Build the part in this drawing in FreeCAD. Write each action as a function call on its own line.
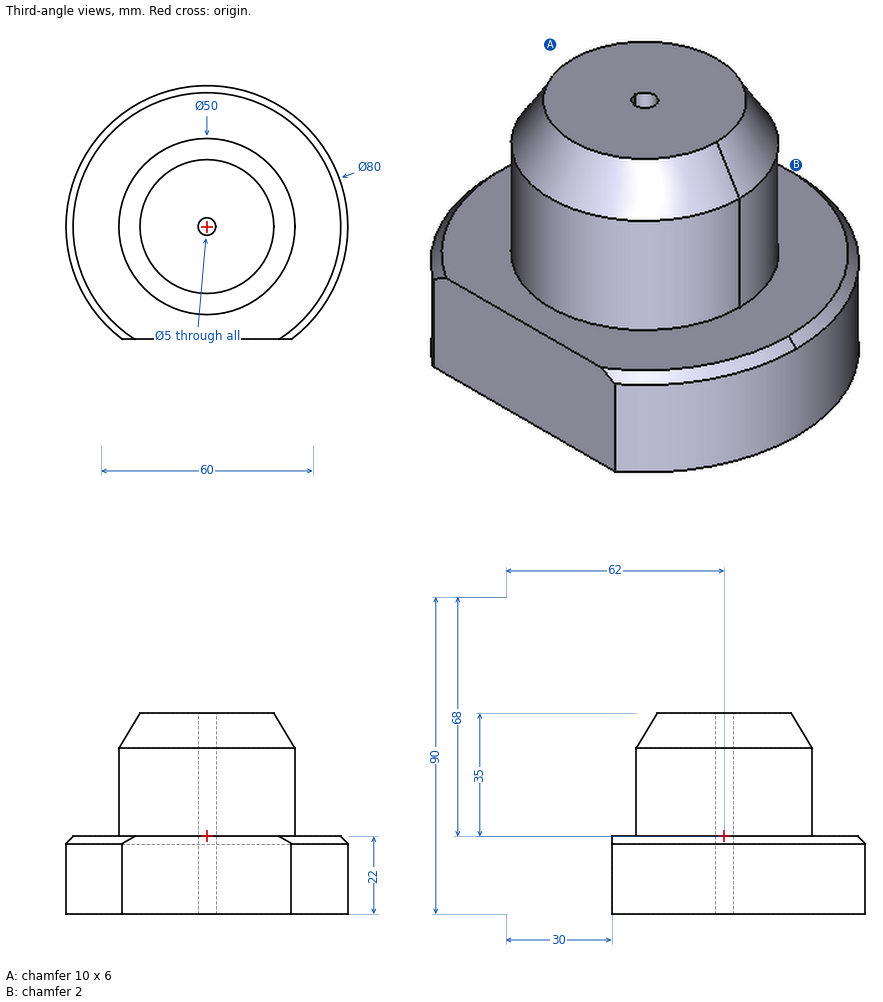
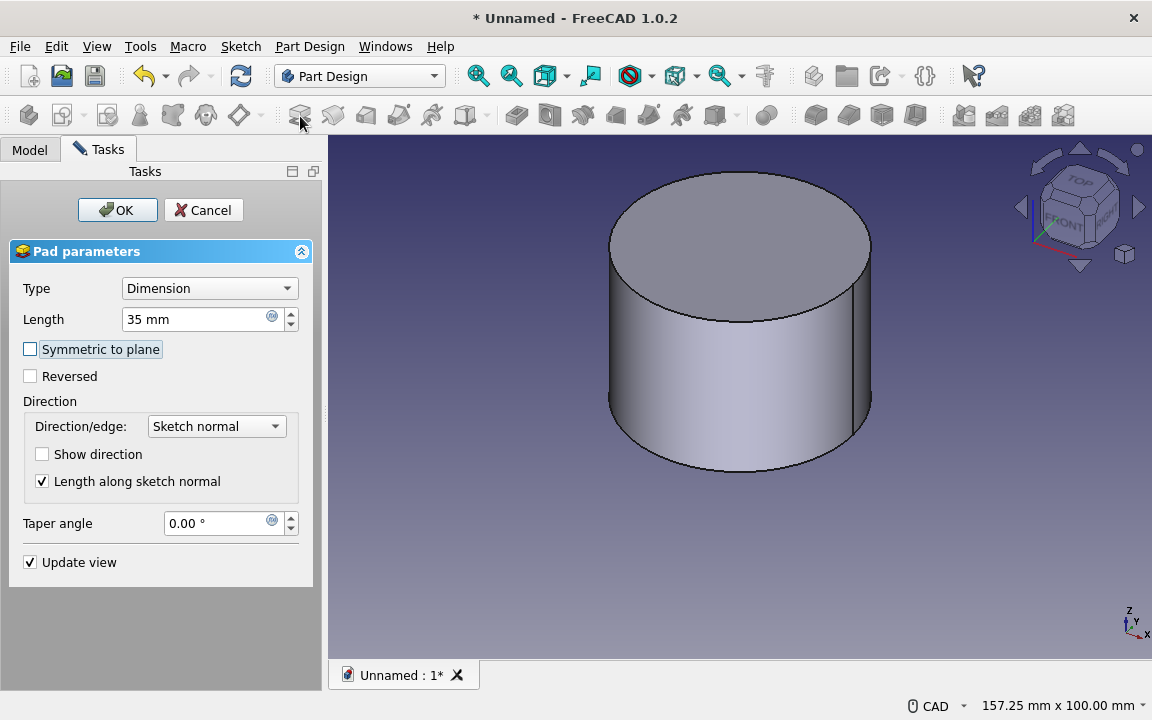
click(118, 210)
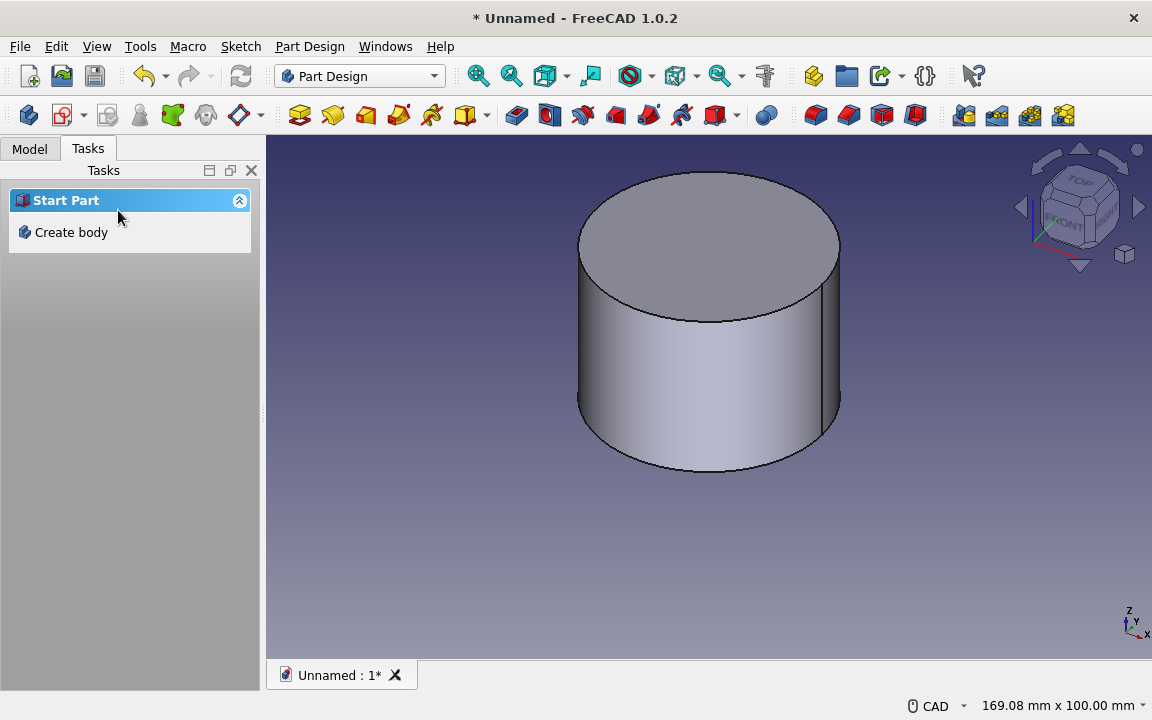
click(579, 254)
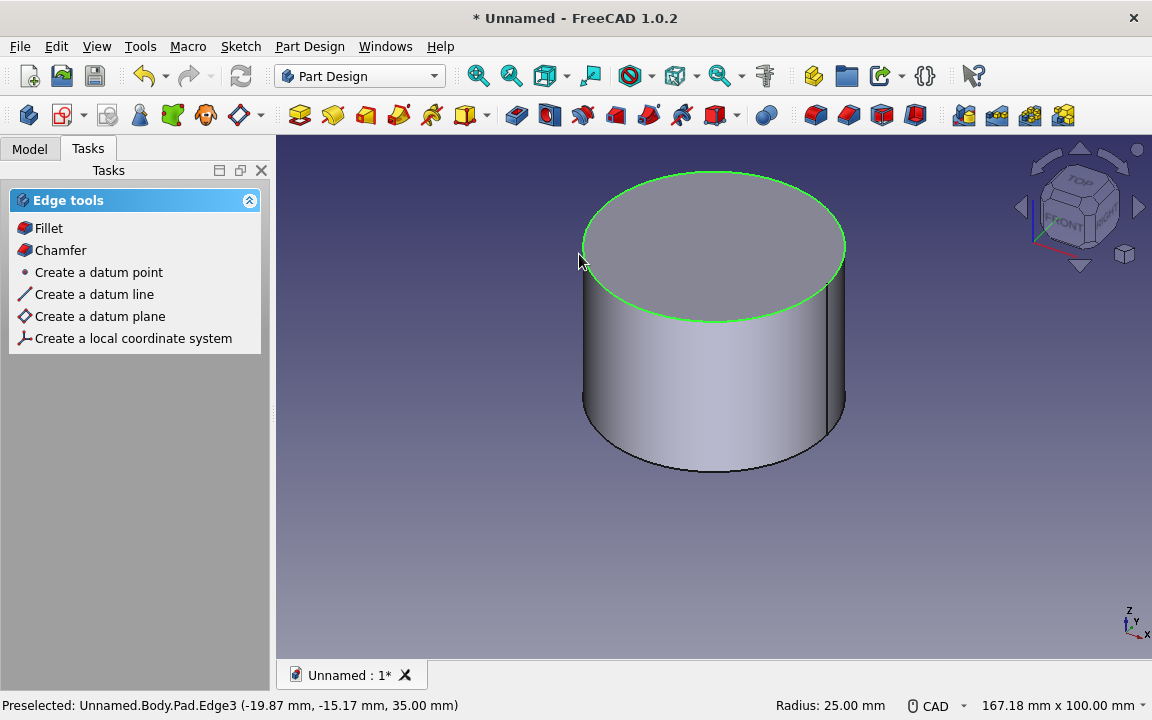
click(849, 116)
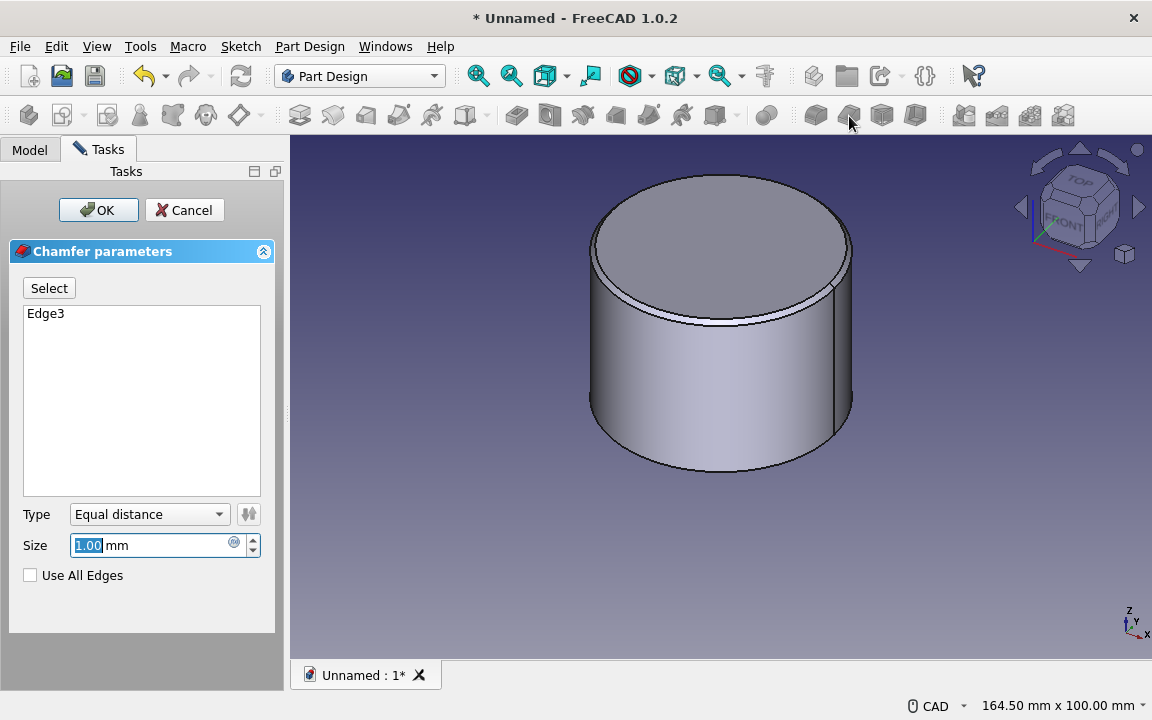
text(10)
key(Tab)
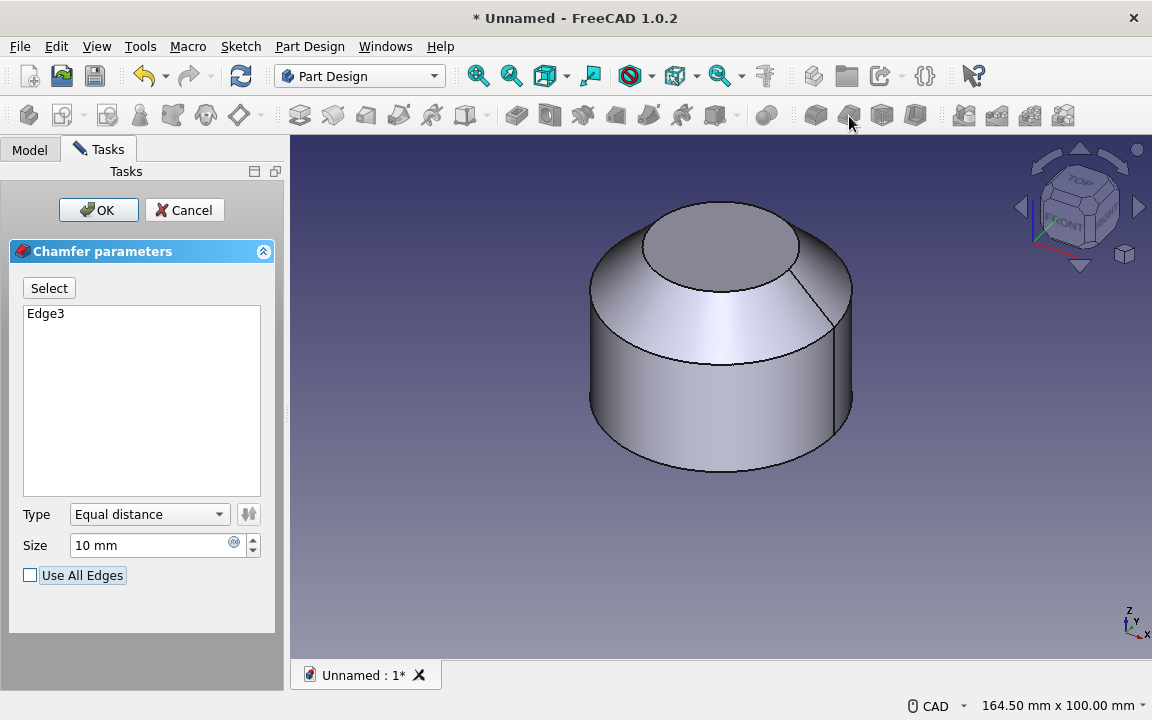
click(150, 514)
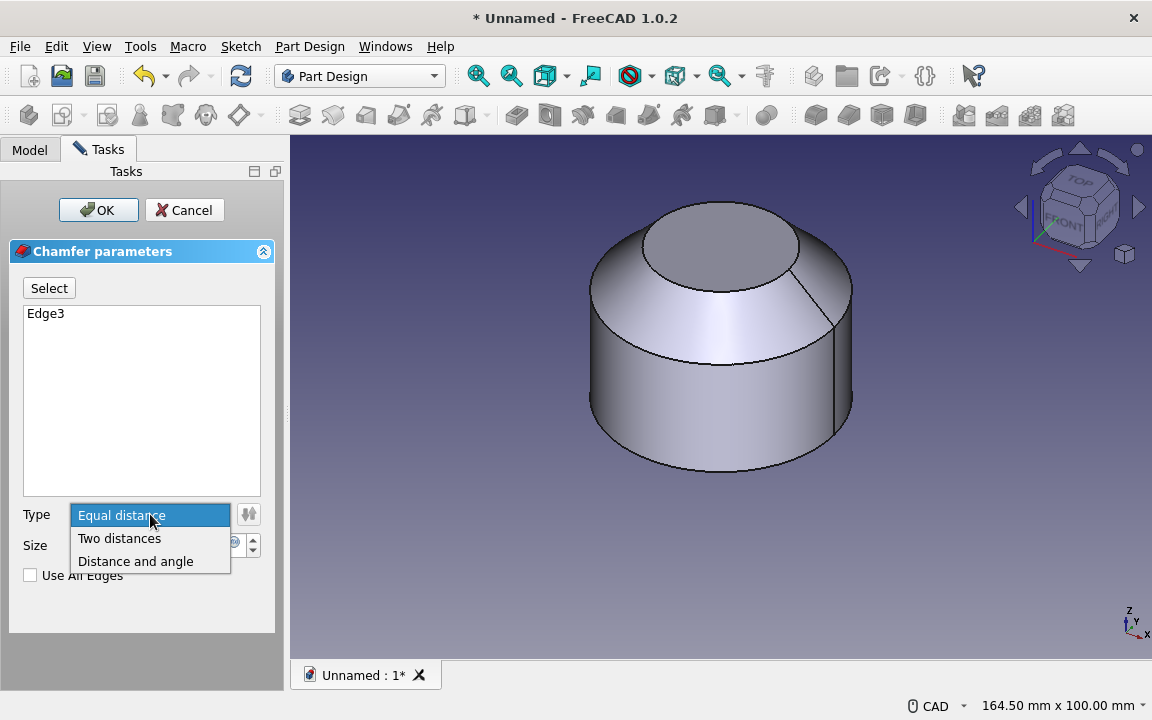
click(148, 538)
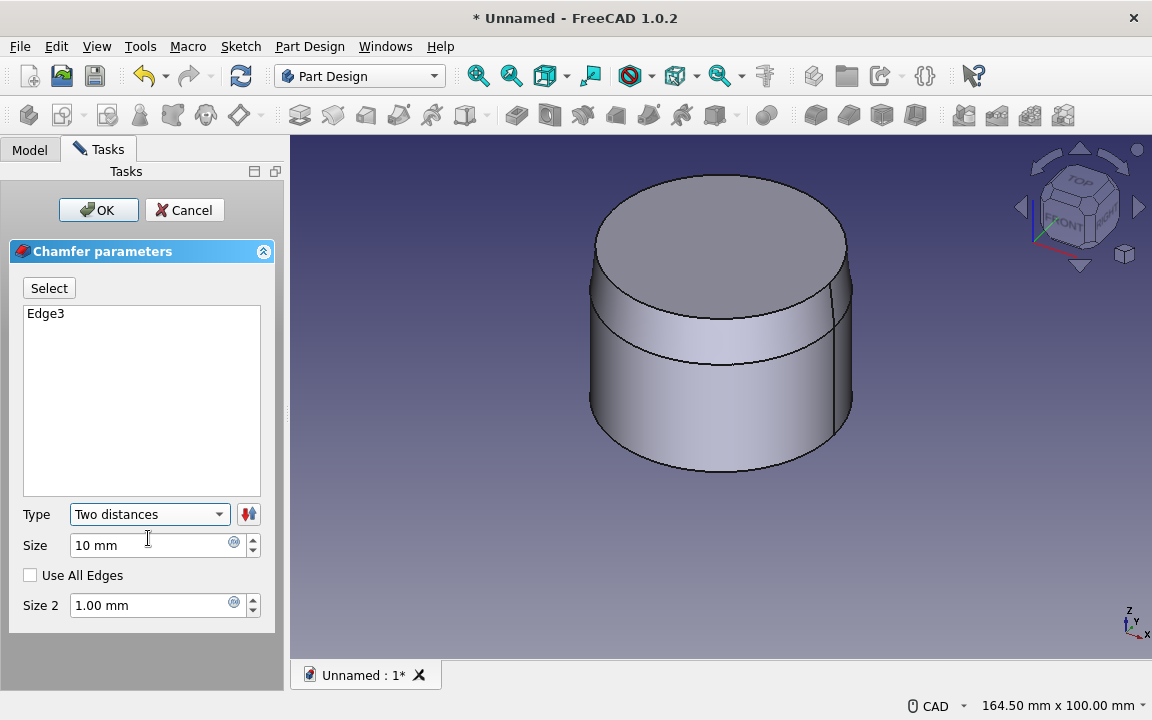
triple_click(158, 606)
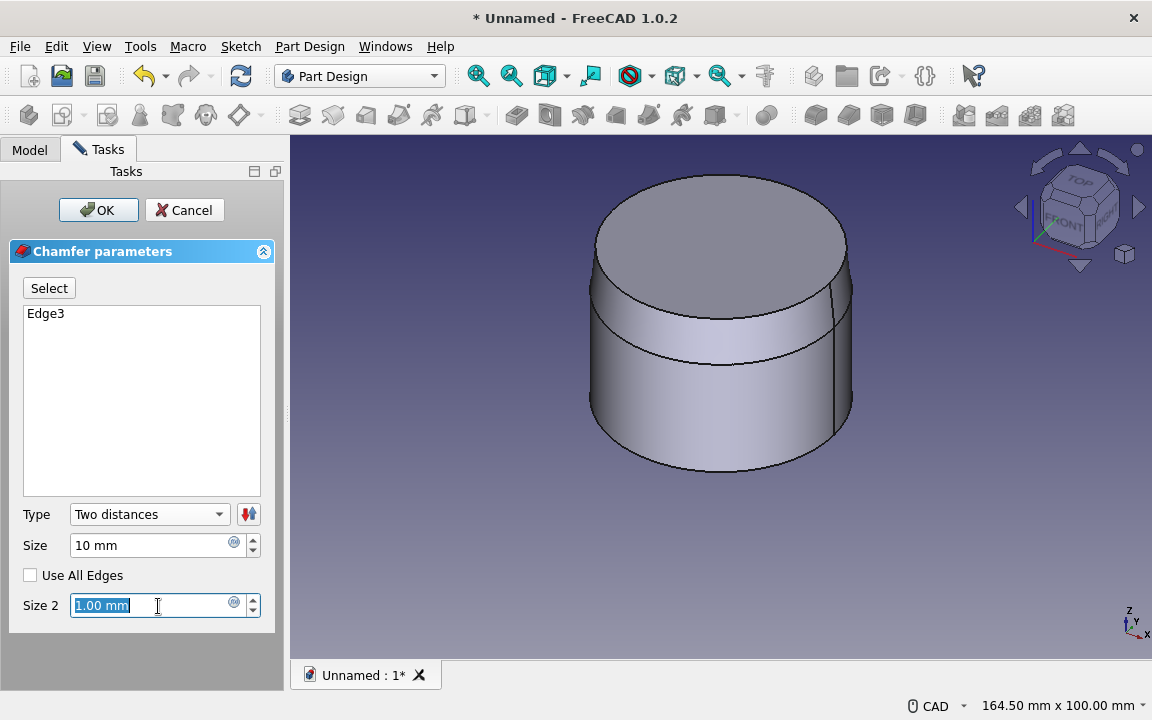
text(6)
key(Tab)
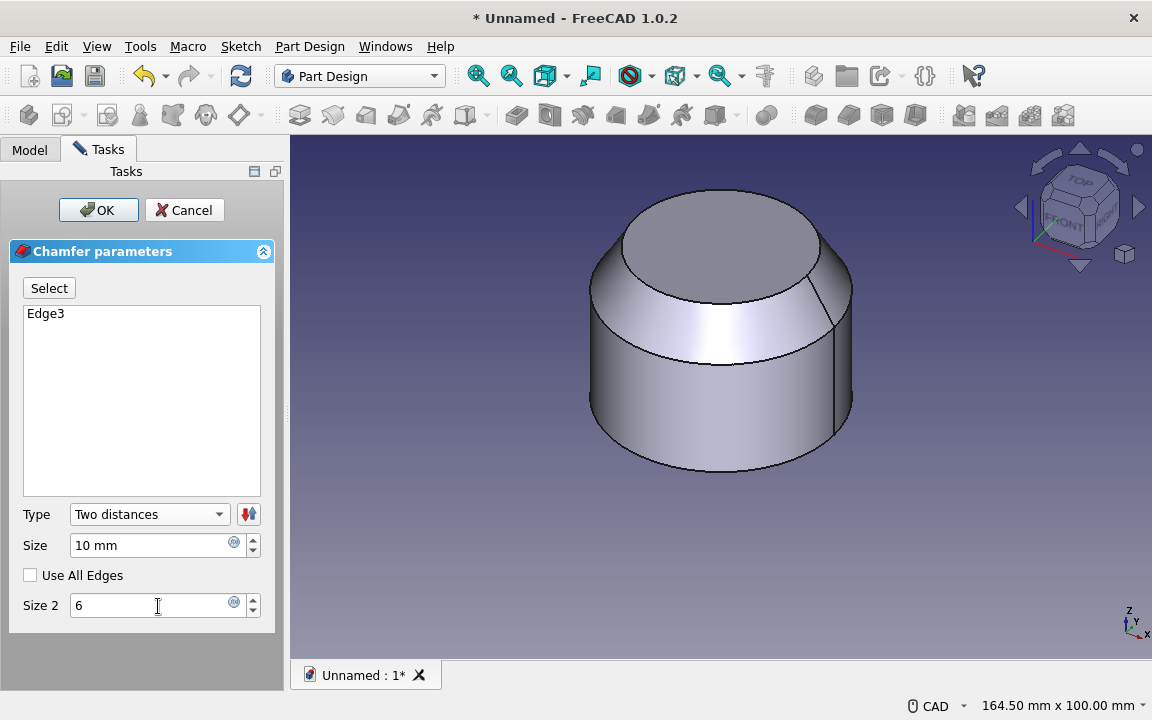
click(99, 210)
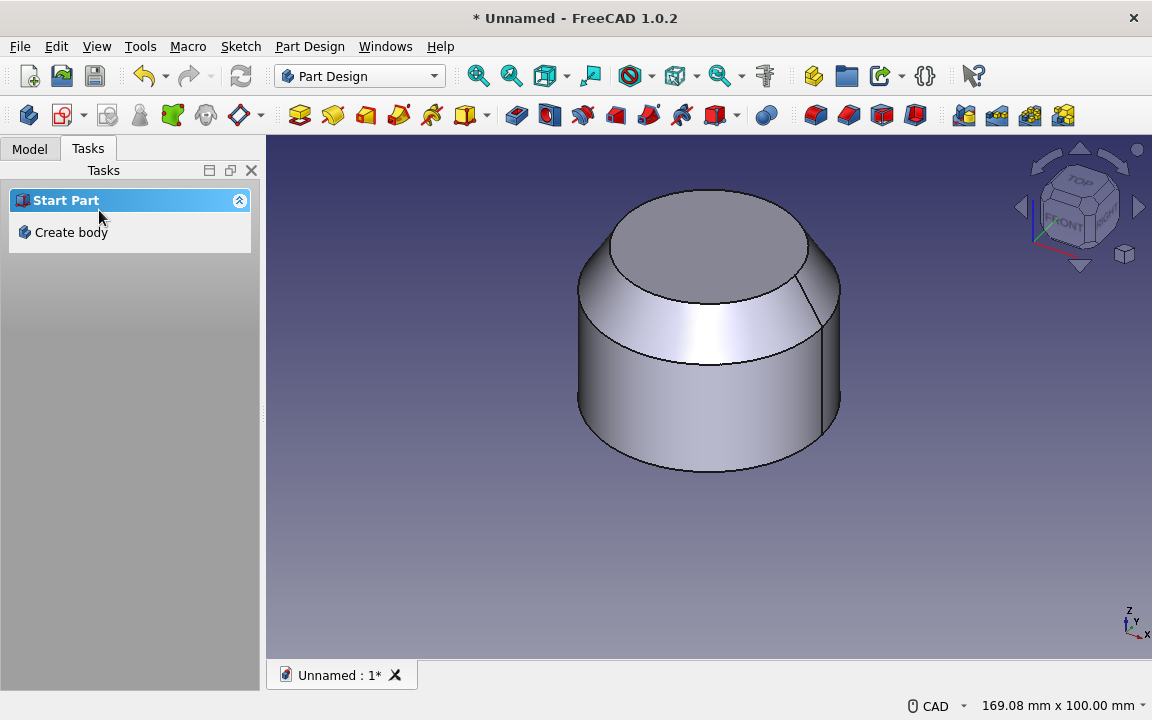
click(62, 116)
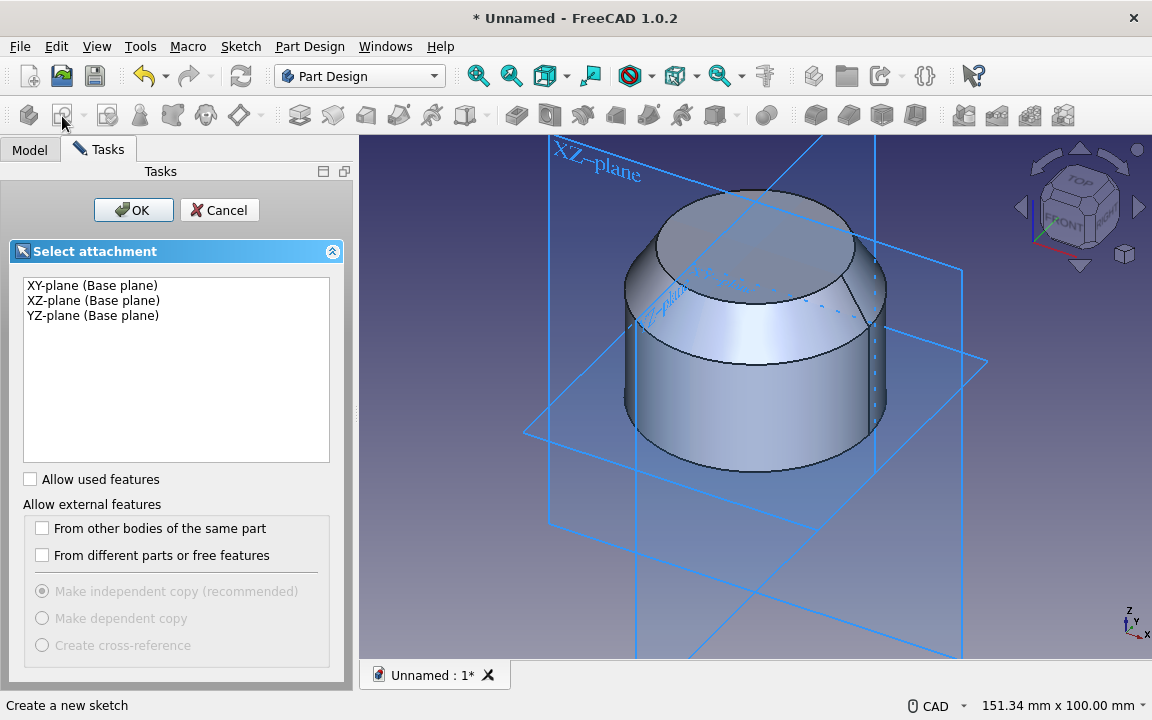
click(84, 286)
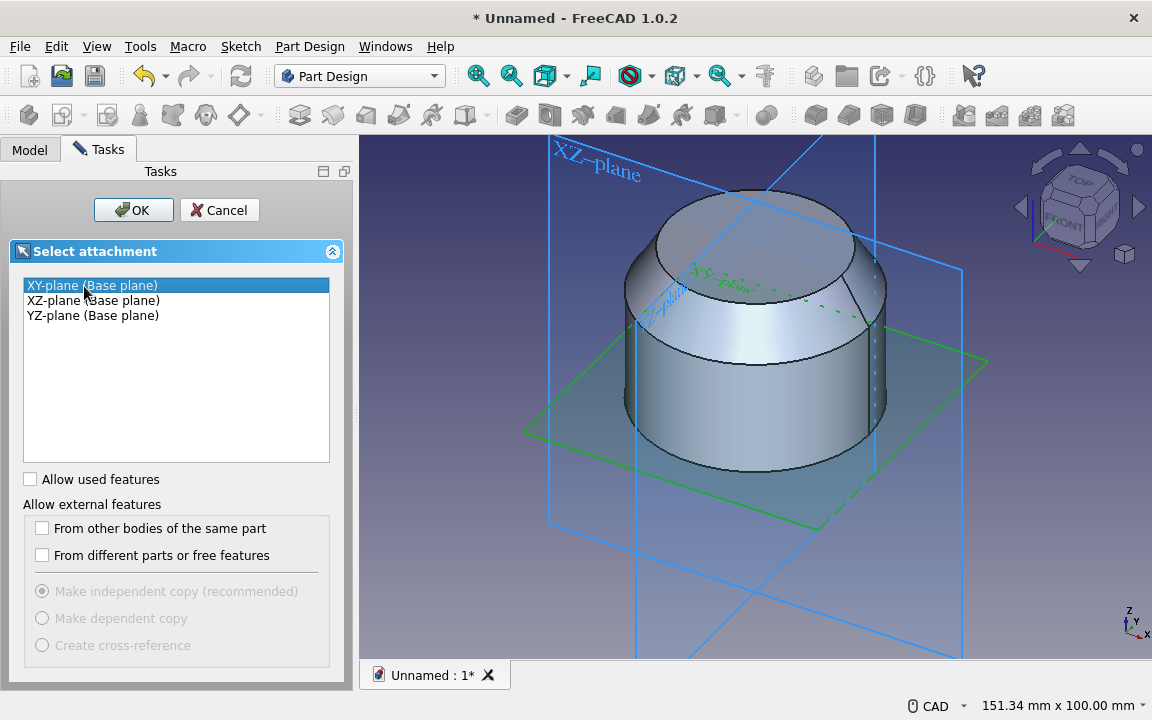
click(134, 210)